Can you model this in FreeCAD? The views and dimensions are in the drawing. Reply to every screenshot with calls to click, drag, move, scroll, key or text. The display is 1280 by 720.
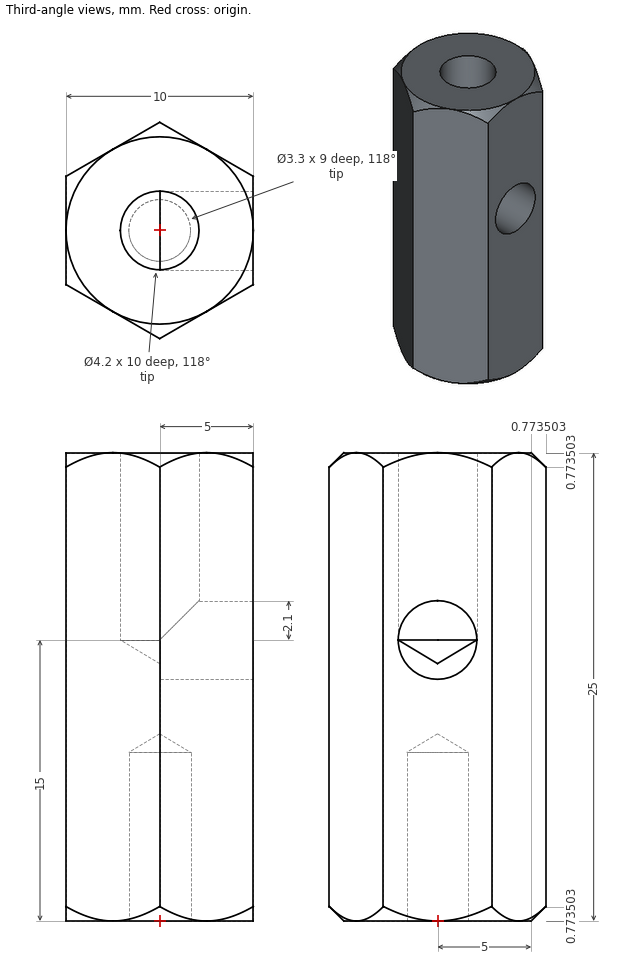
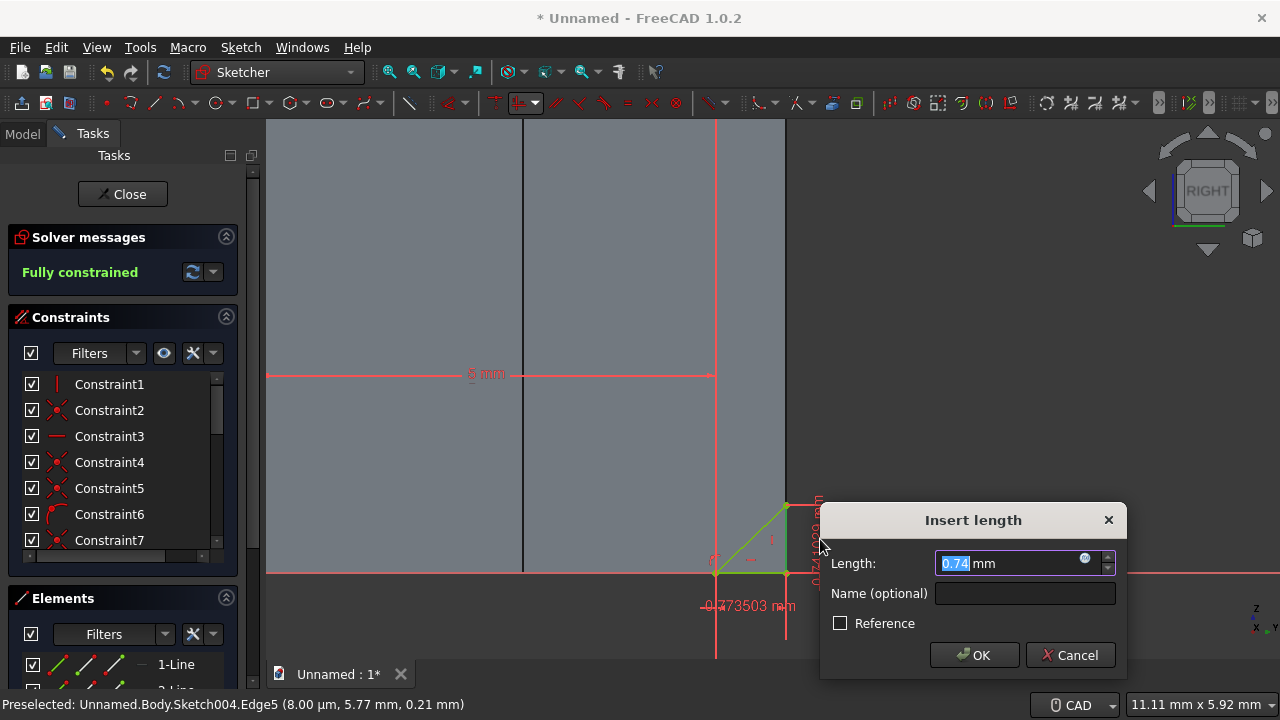
text(0.773503)
key(Return)
key(Escape)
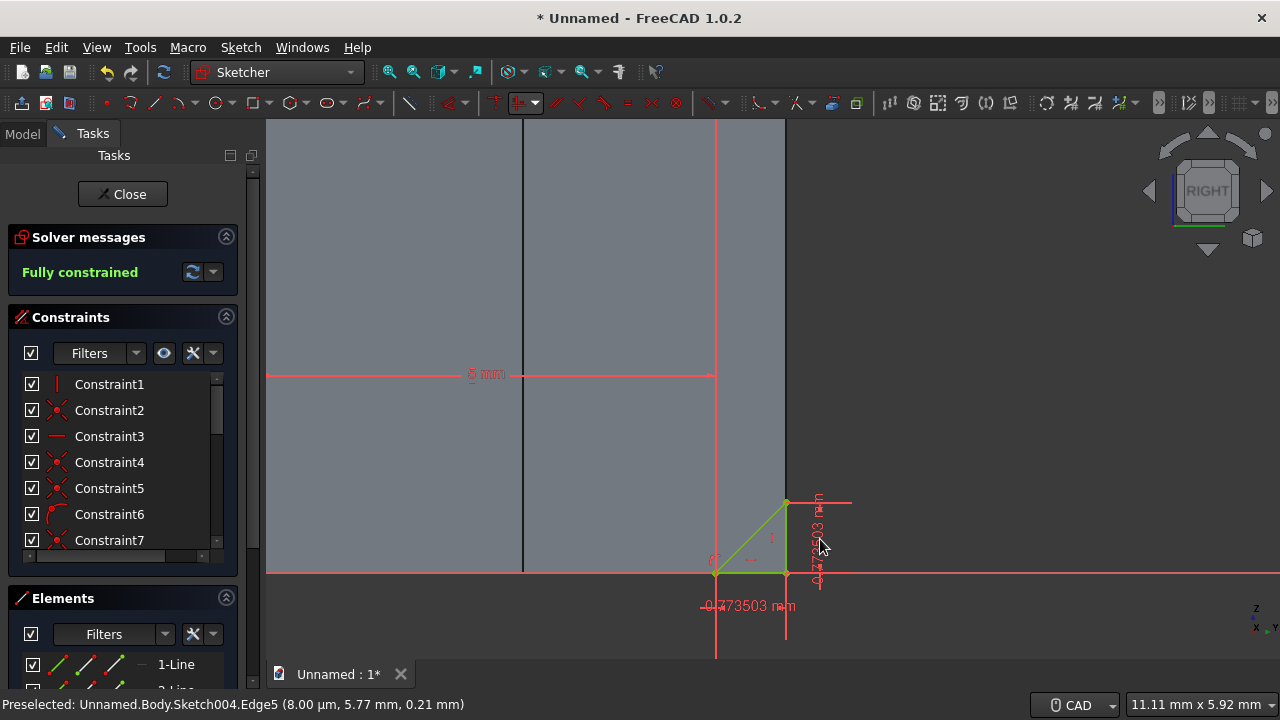
click(123, 194)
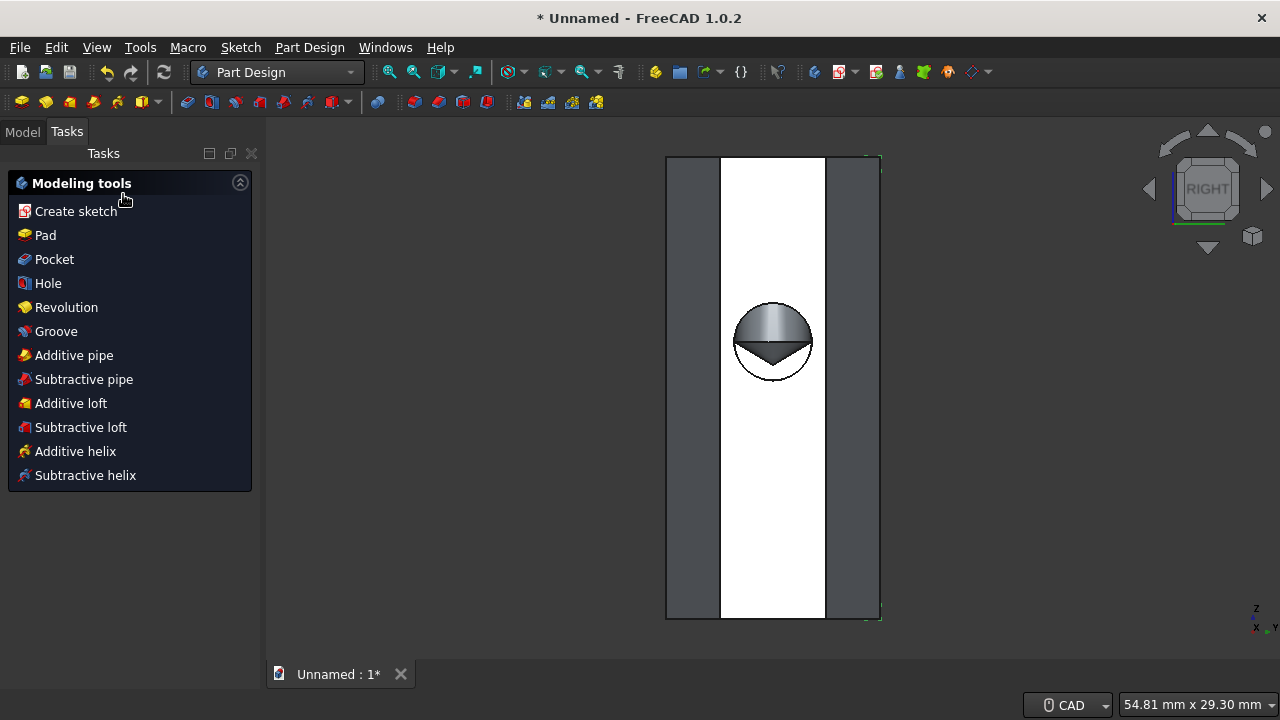
click(236, 102)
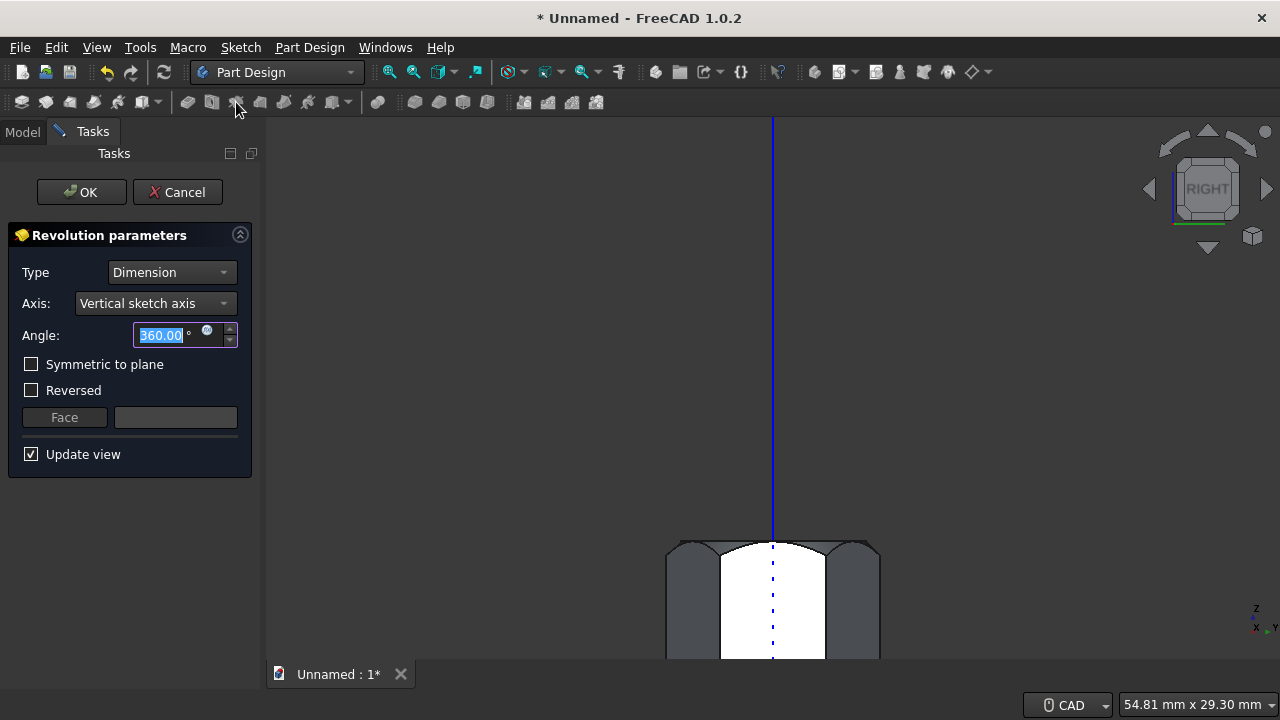
click(82, 192)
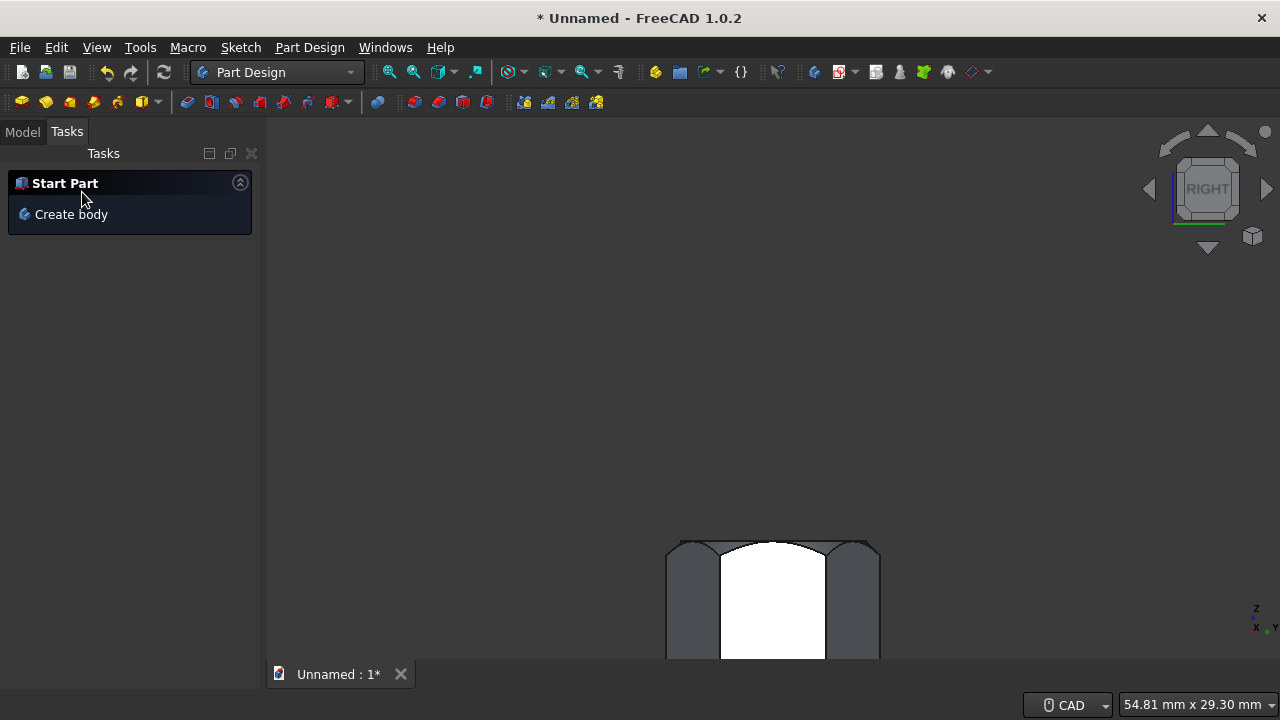
key(0)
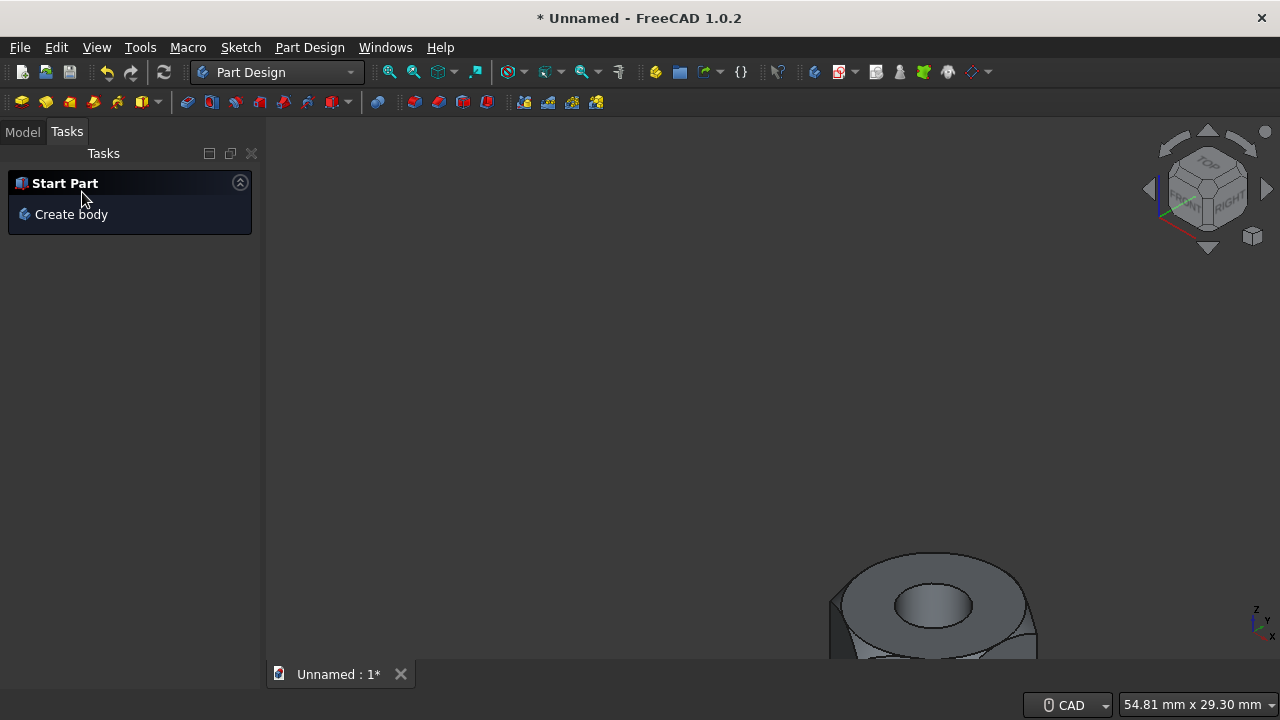
click(390, 72)